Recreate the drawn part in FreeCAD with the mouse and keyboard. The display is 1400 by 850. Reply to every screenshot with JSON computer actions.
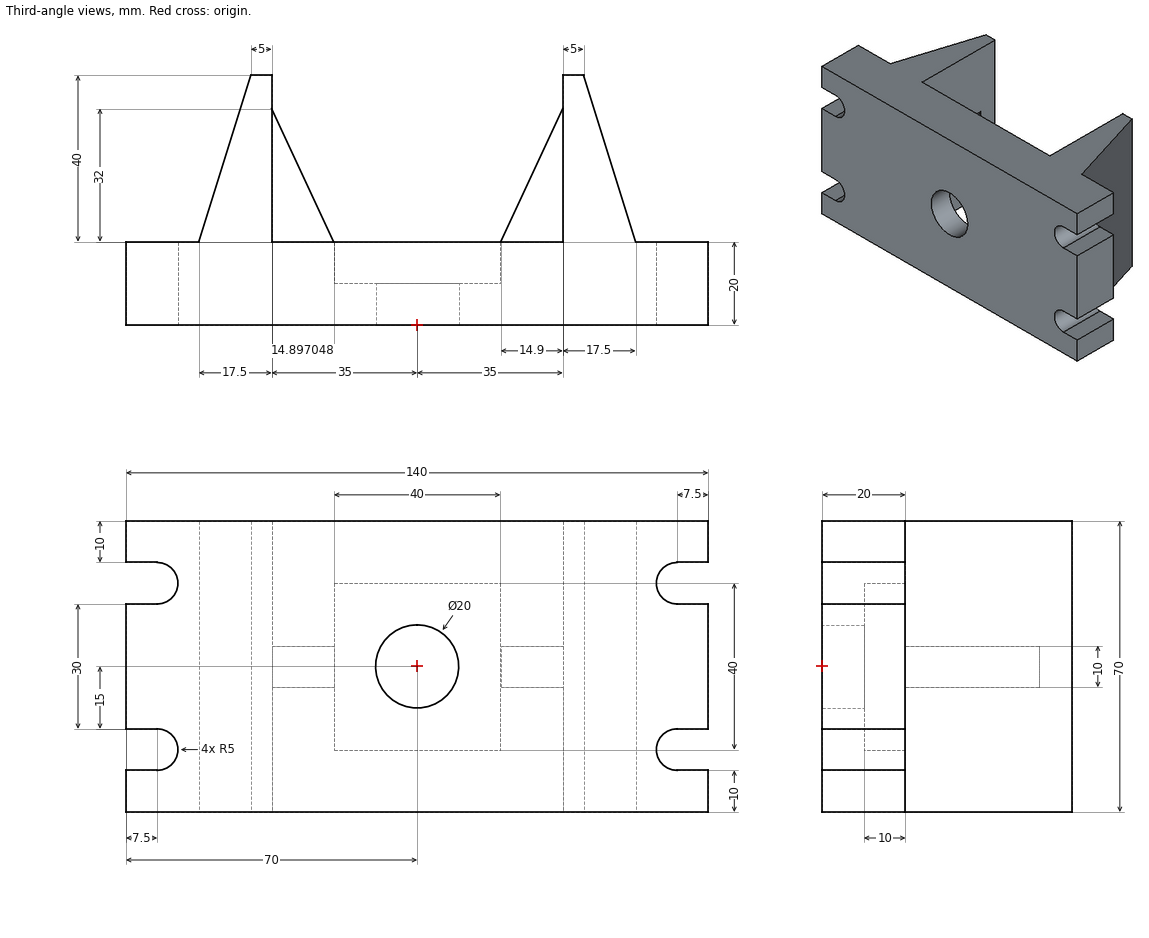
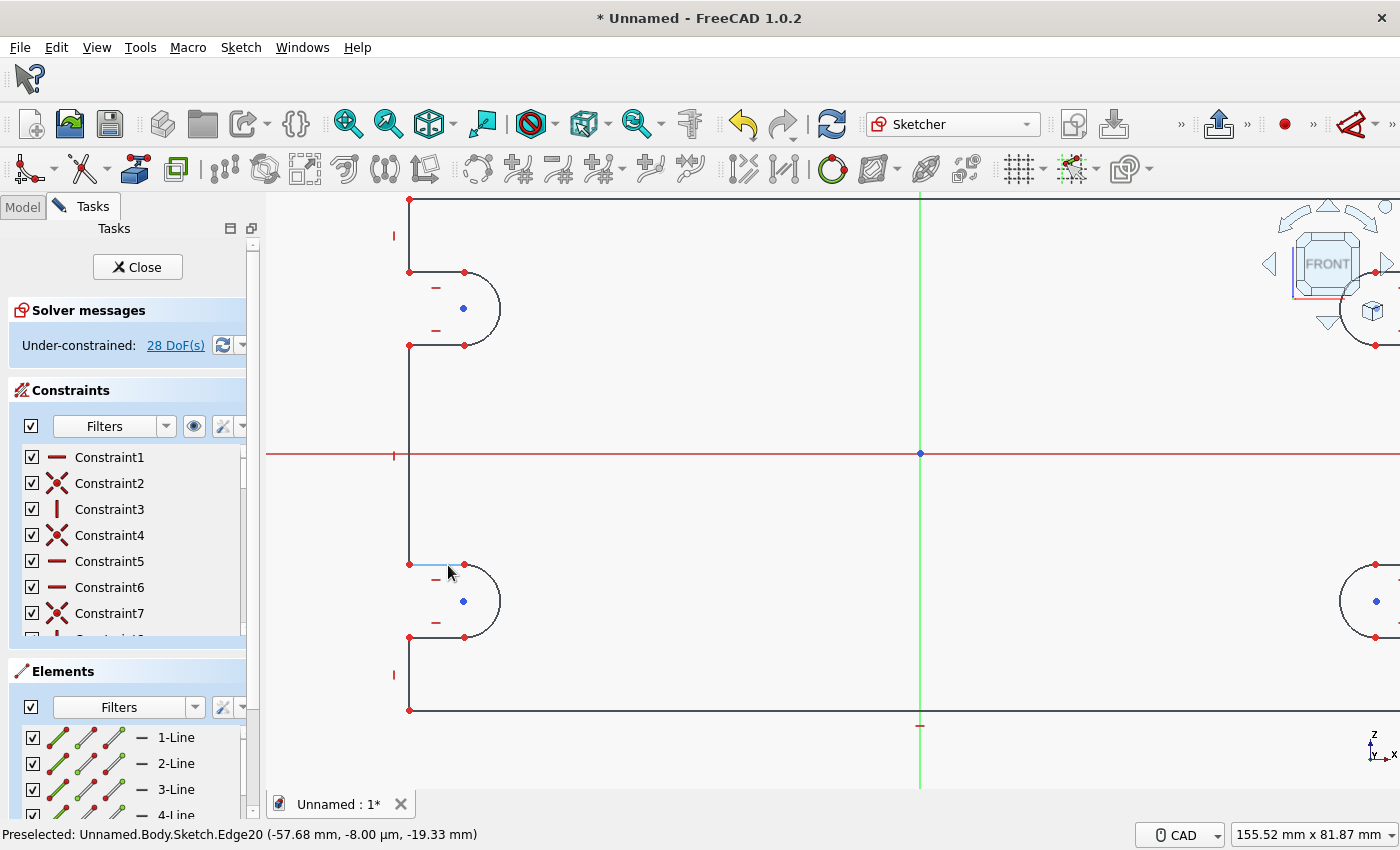
{"action": "left_click", "coordinate": [448, 565]}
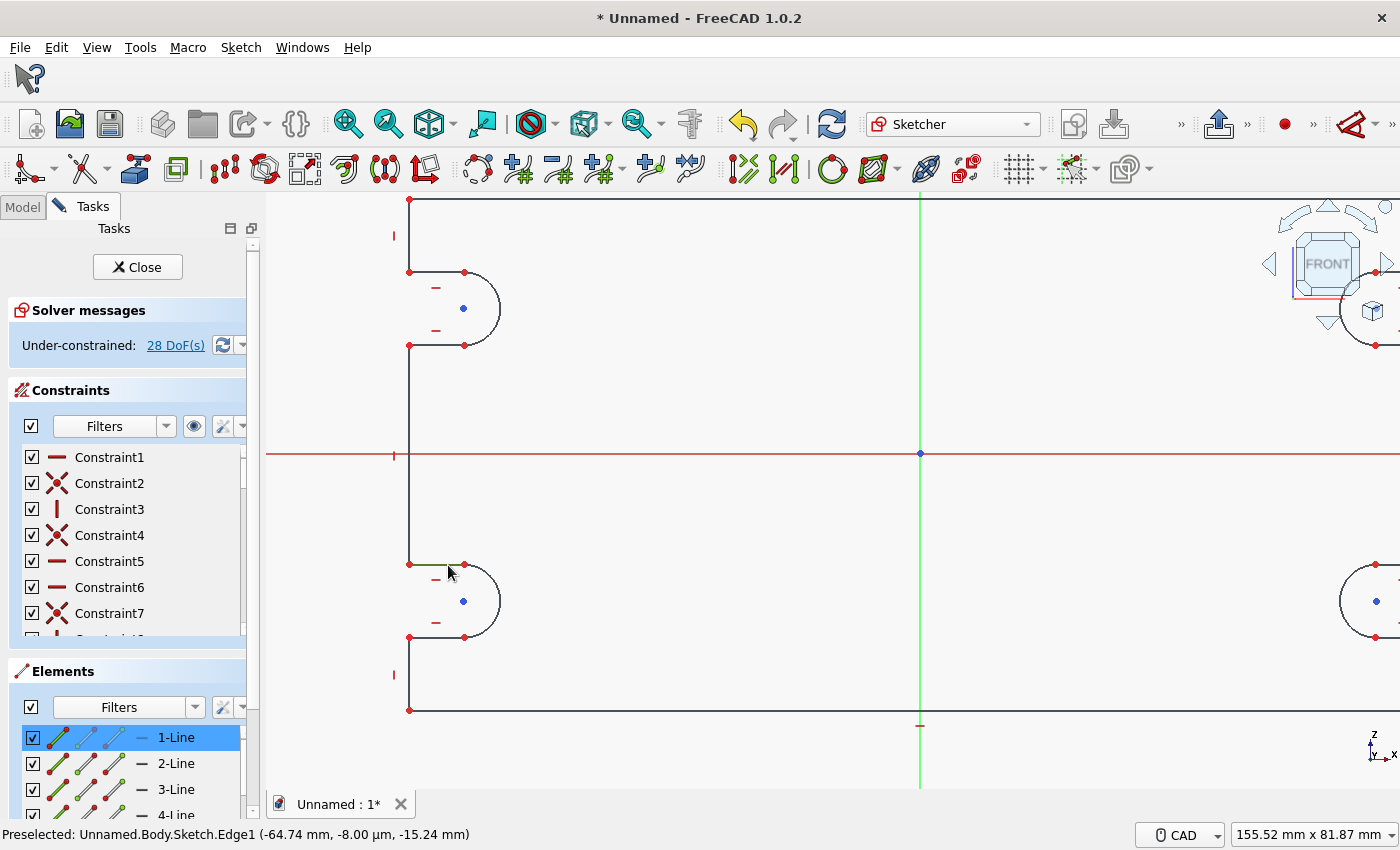
{"action": "left_click", "coordinate": [493, 622]}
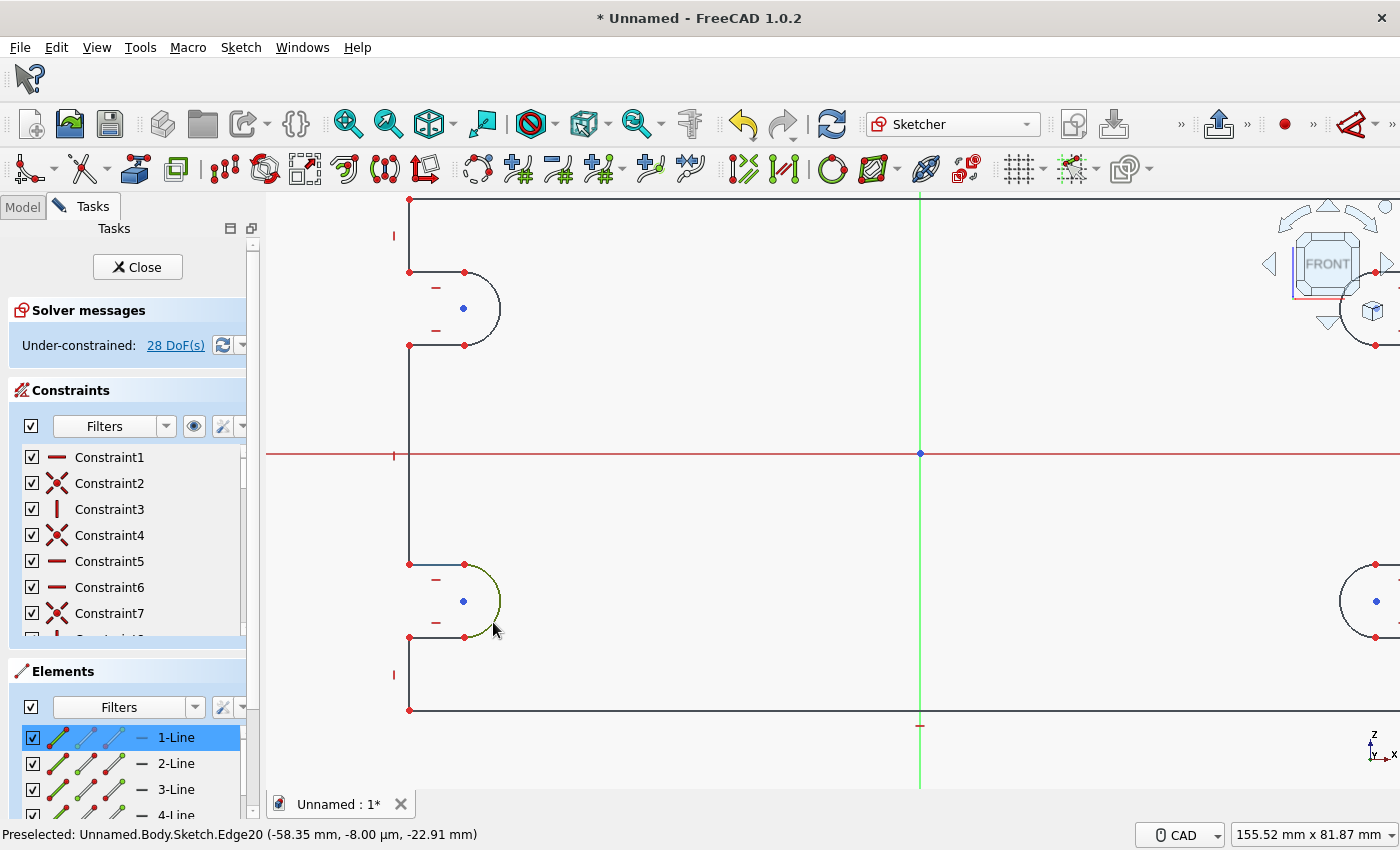
{"action": "key", "text": "t"}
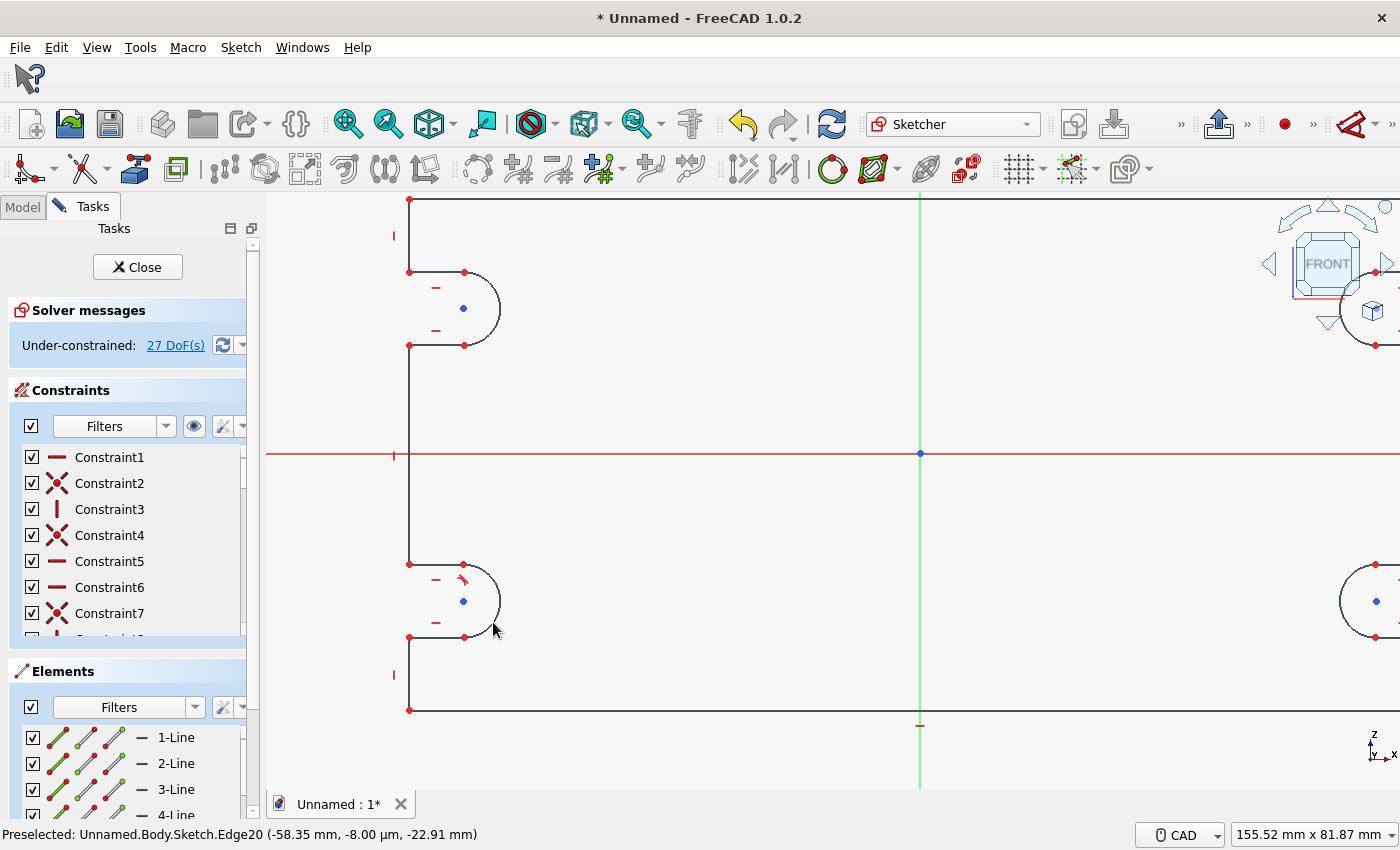
{"action": "left_click", "coordinate": [426, 345]}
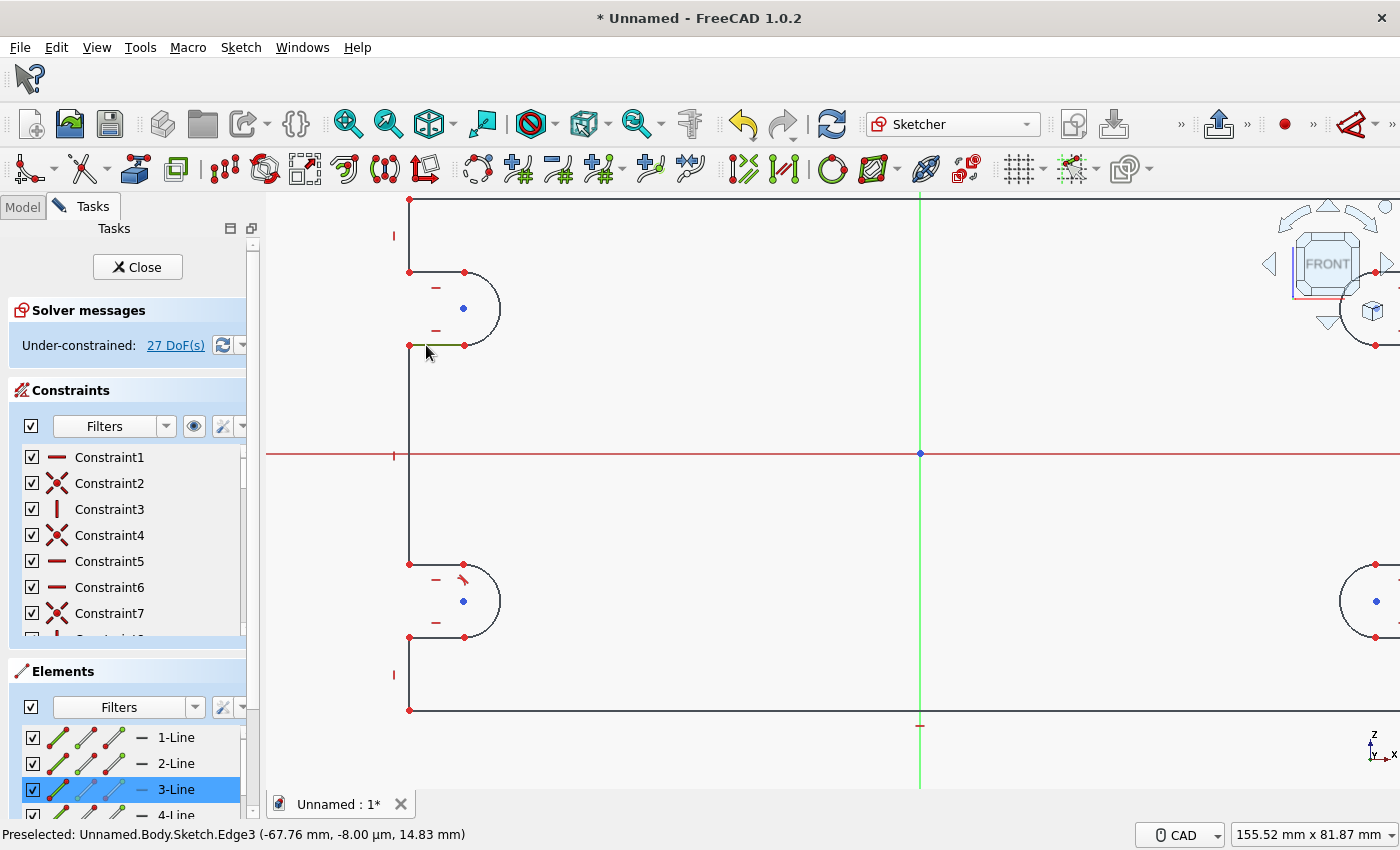
{"action": "left_click", "coordinate": [493, 330]}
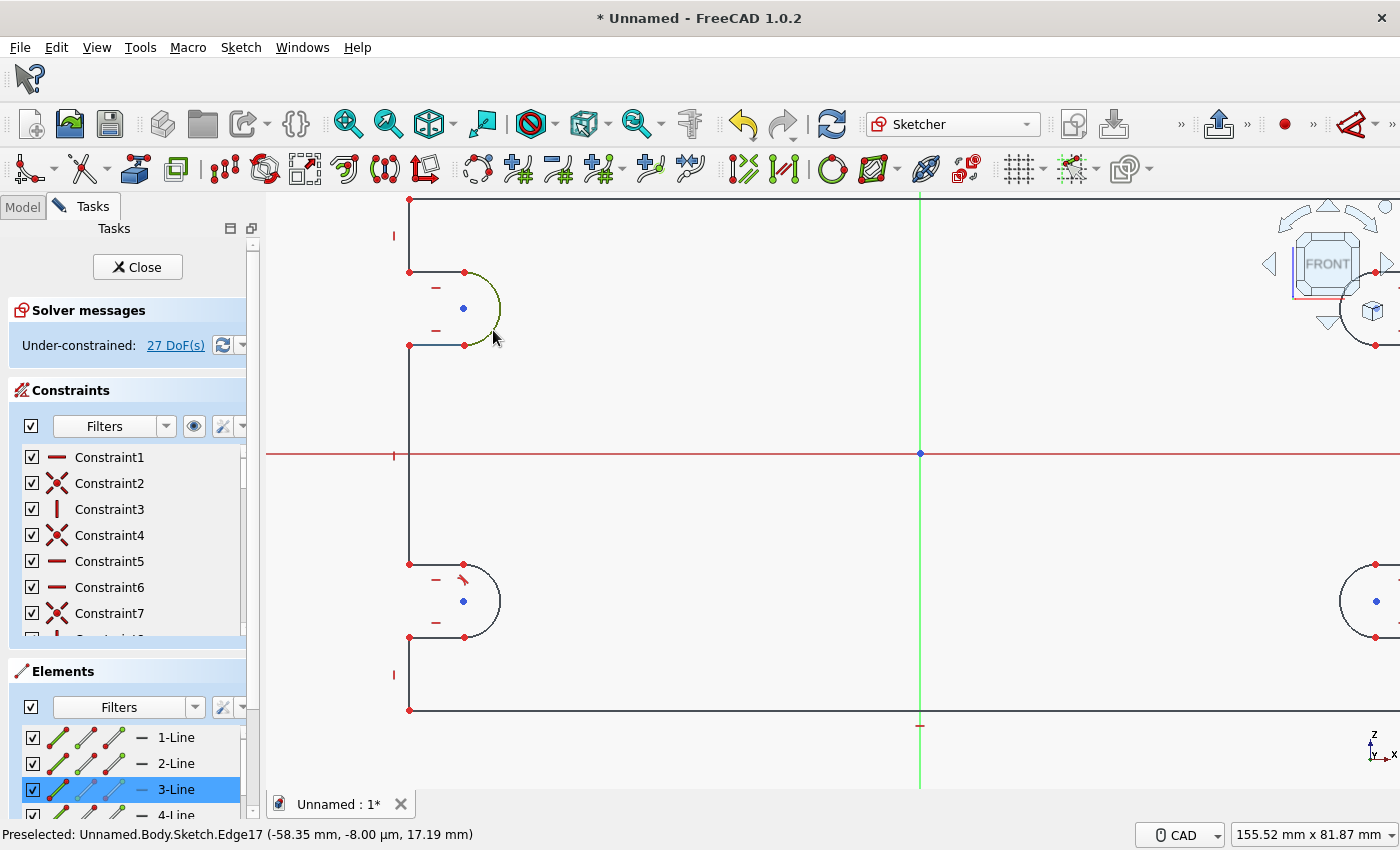
{"action": "key", "text": "t"}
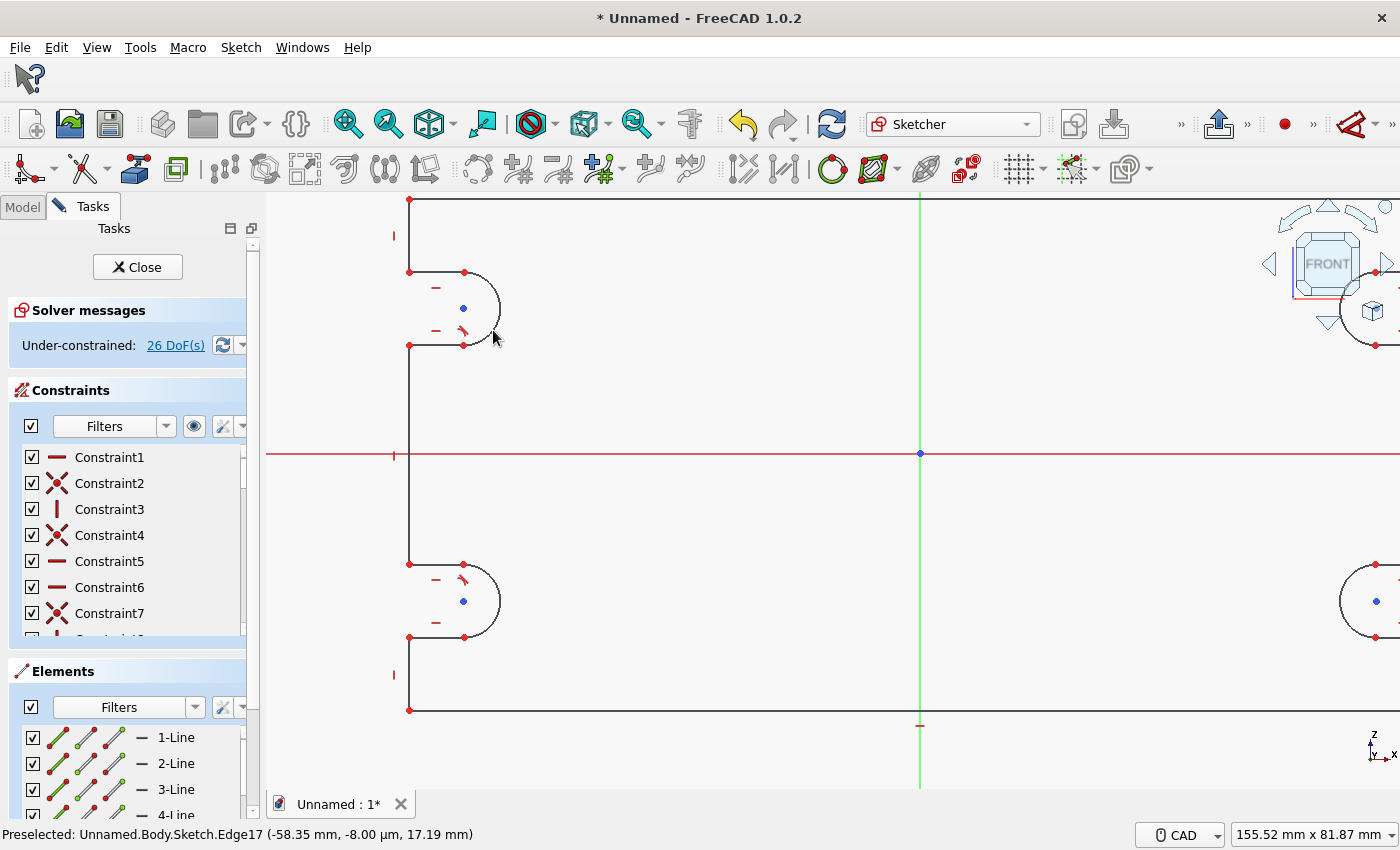
{"action": "left_click", "coordinate": [448, 272]}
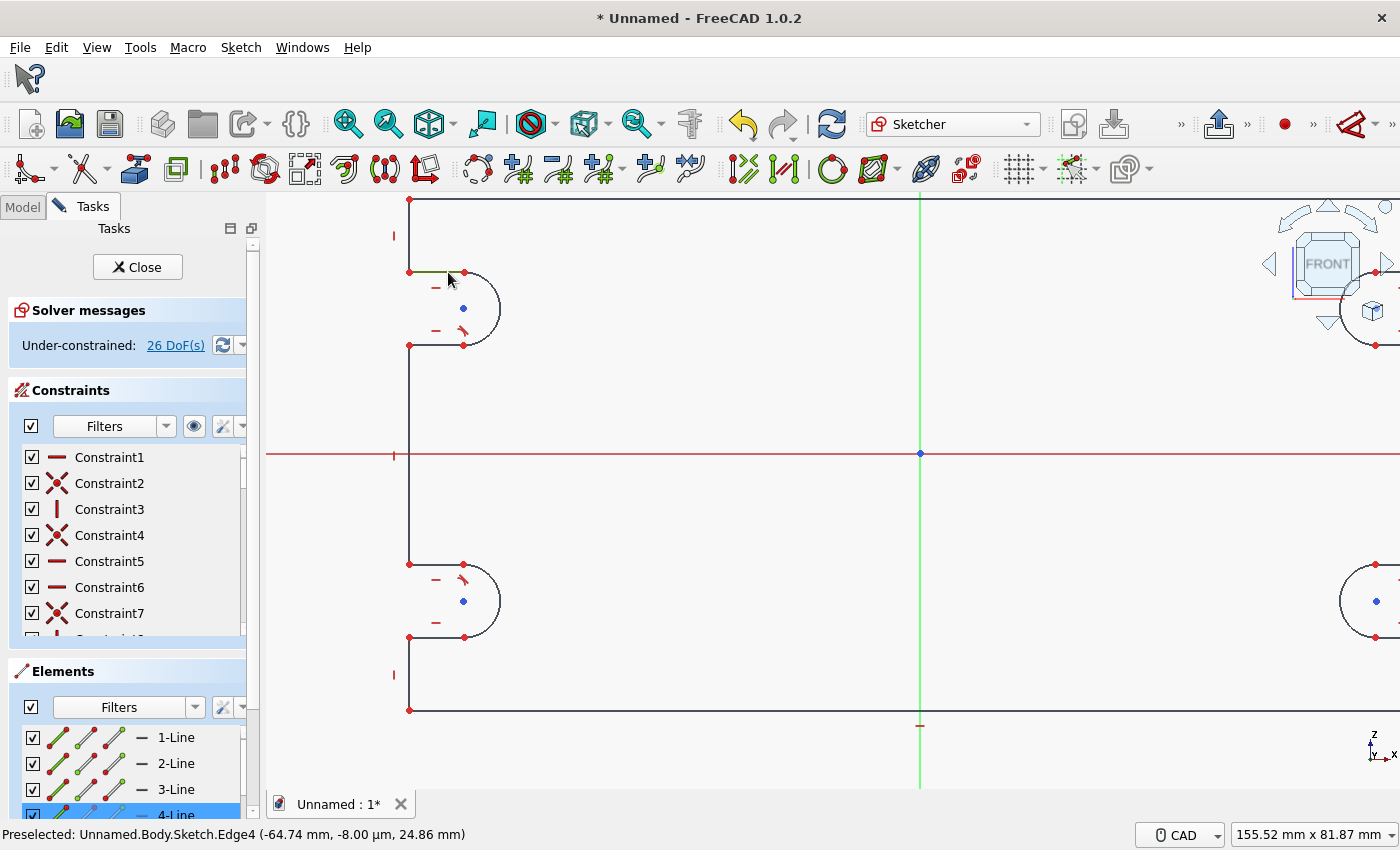
{"action": "left_click", "coordinate": [493, 331]}